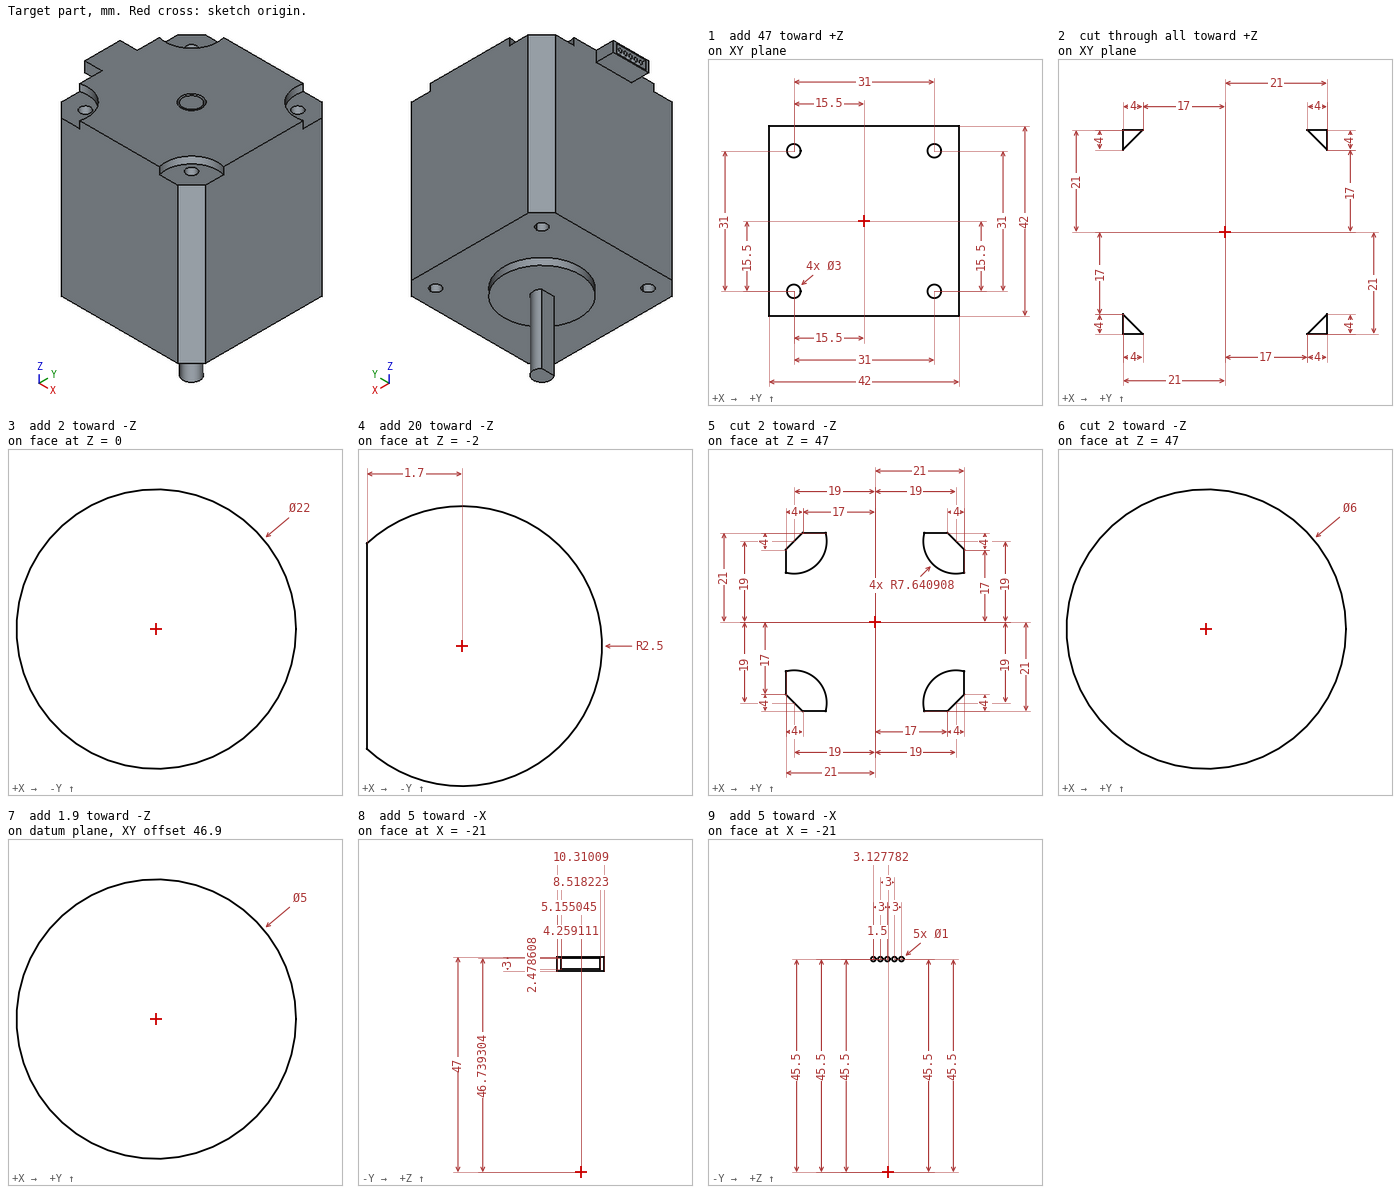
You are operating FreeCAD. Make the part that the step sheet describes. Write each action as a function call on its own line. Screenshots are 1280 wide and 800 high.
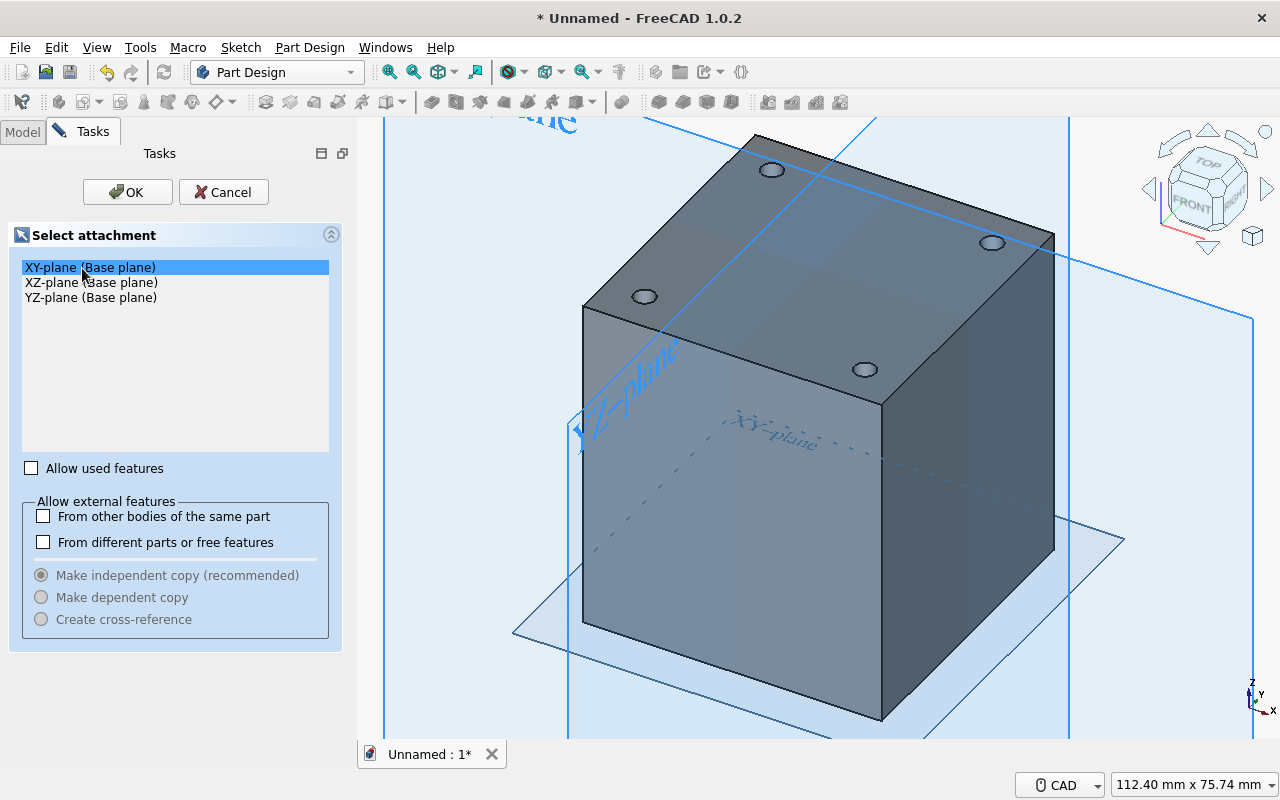
click(128, 192)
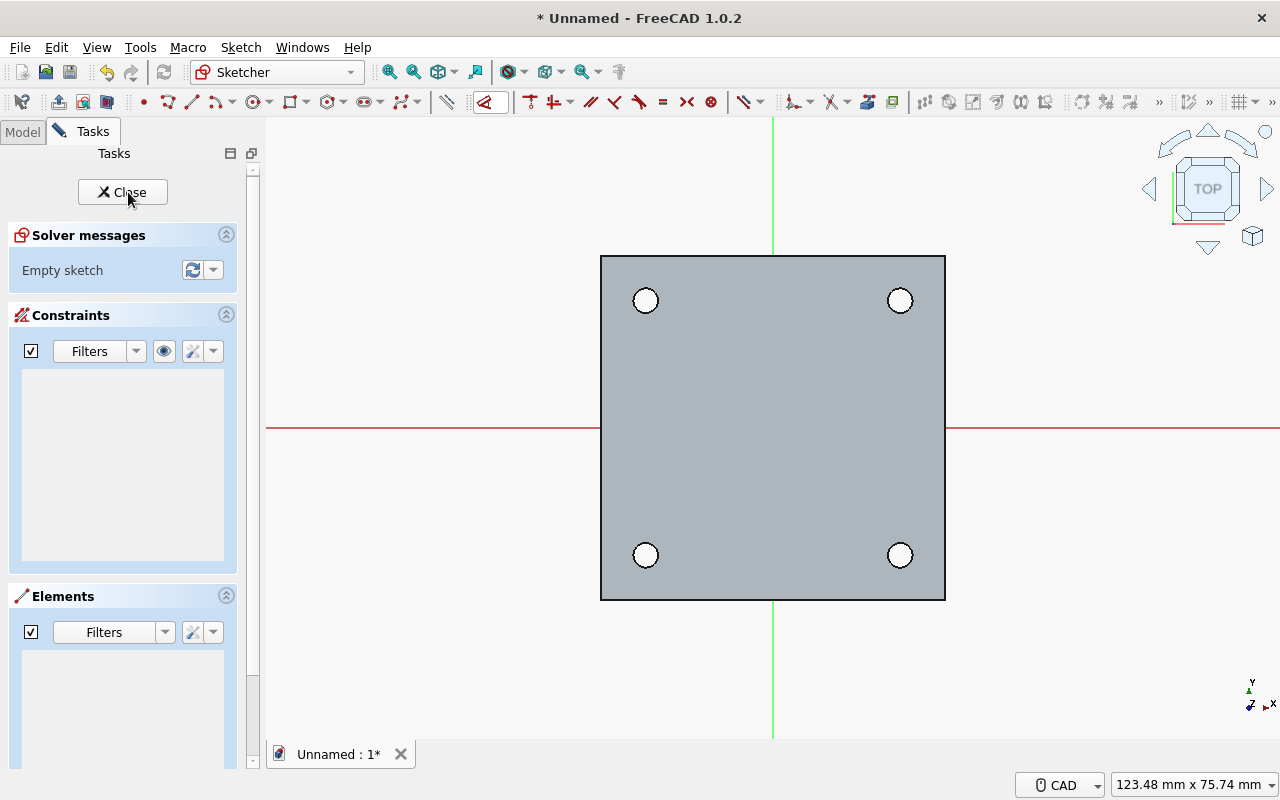
click(108, 102)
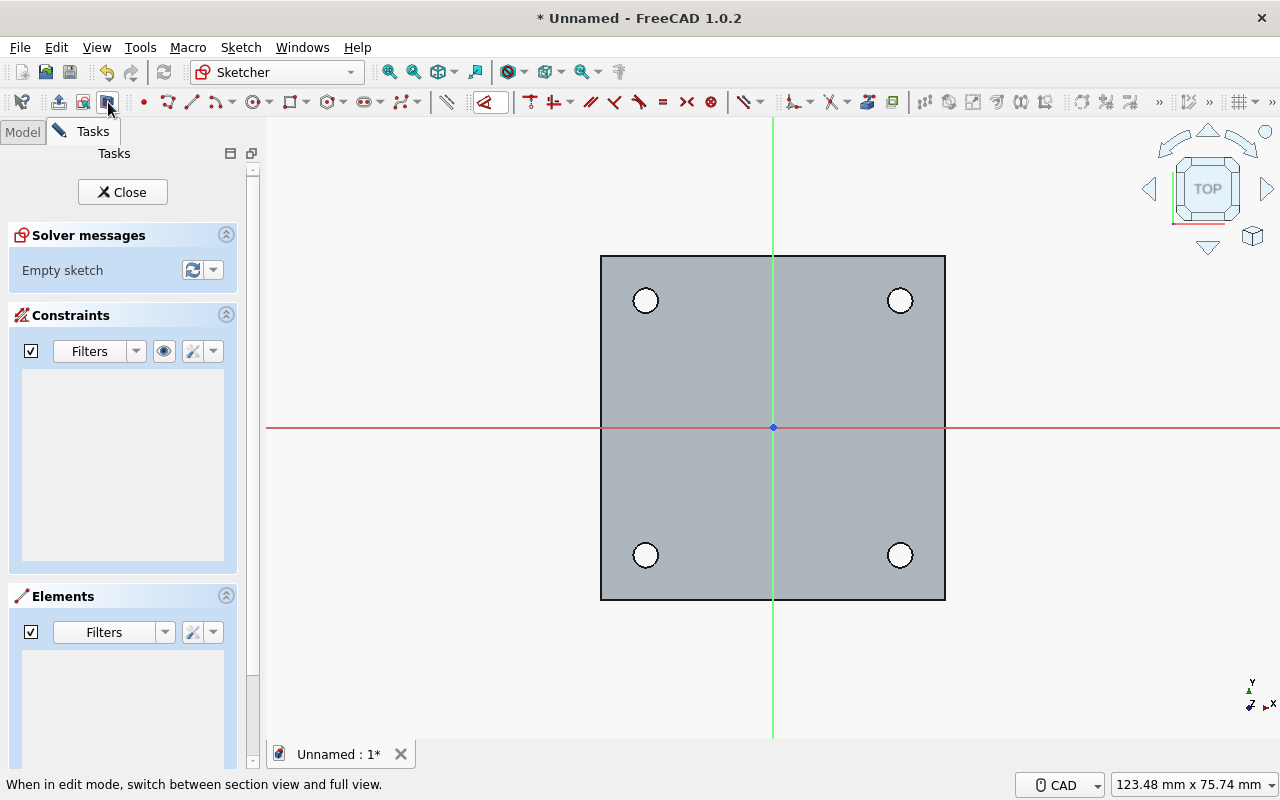
click(168, 102)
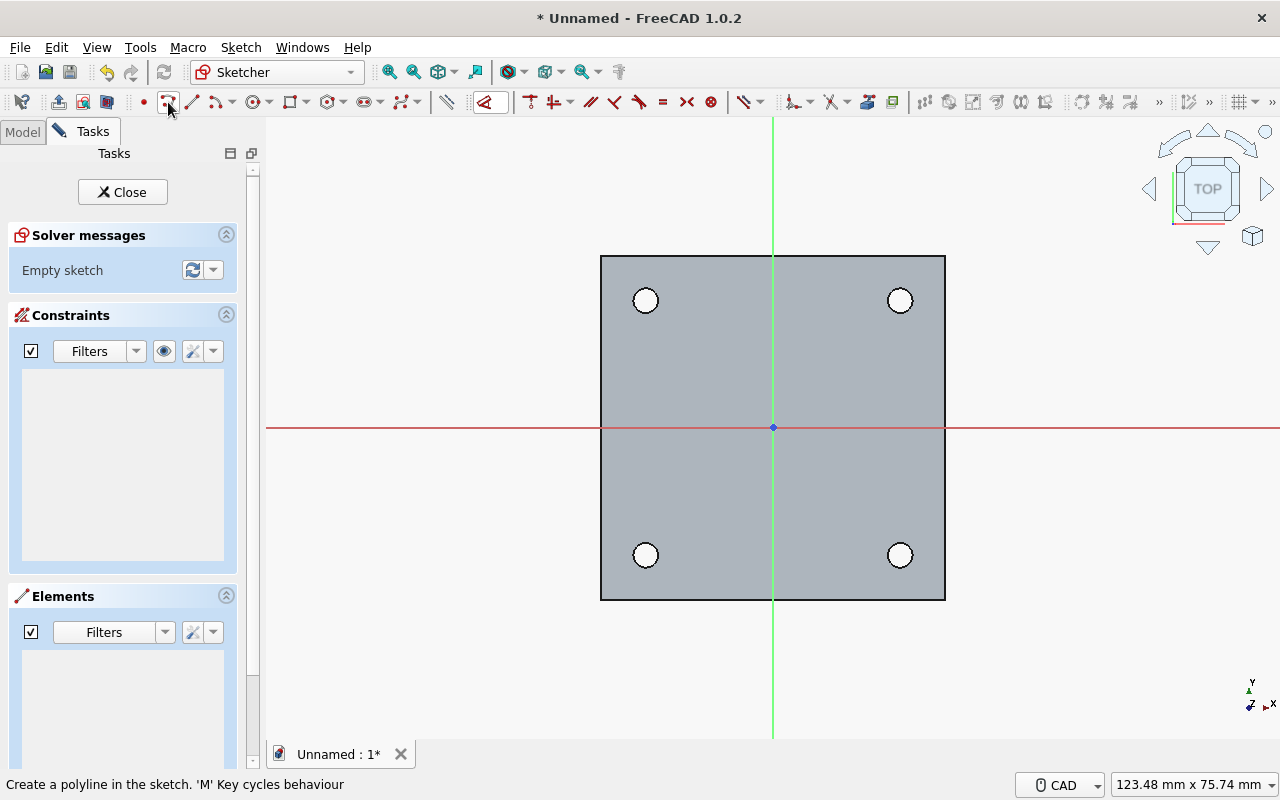
click(945, 288)
click(913, 256)
click(945, 256)
click(945, 289)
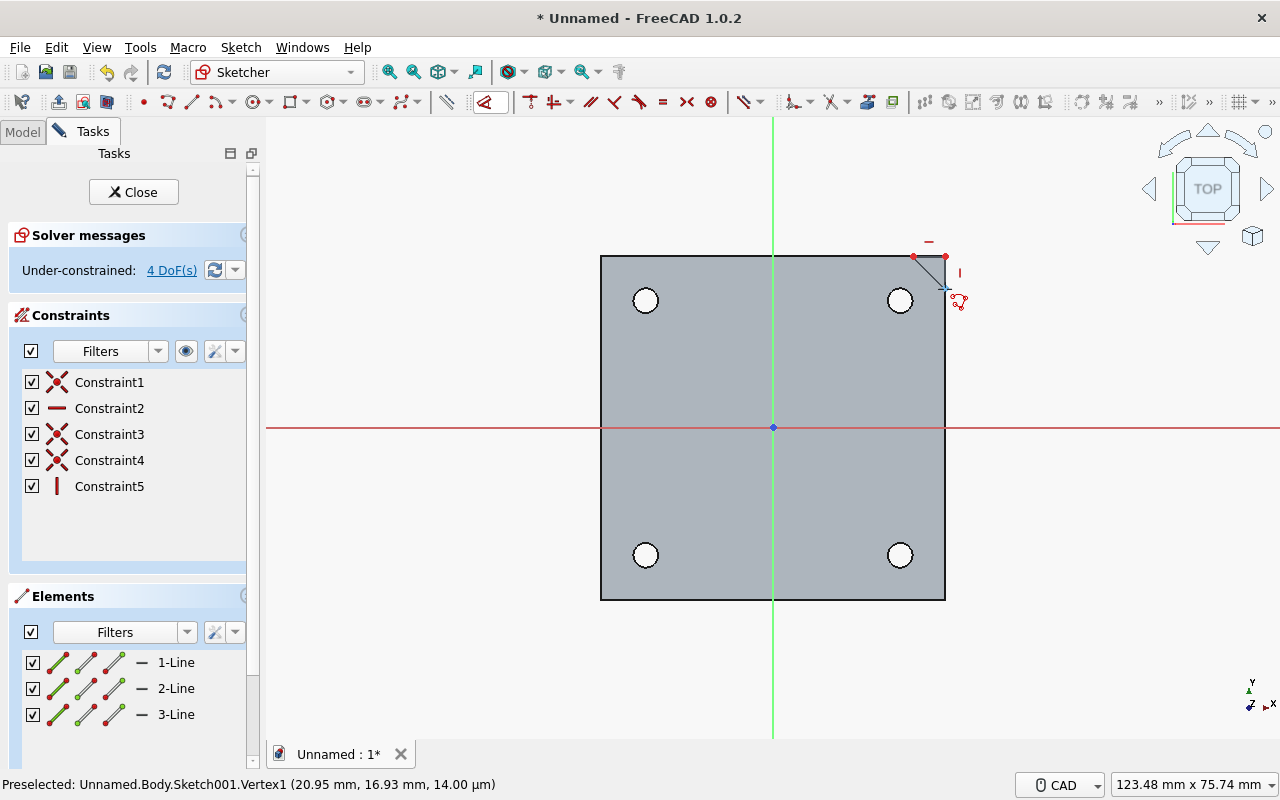
click(633, 256)
click(601, 288)
click(601, 256)
click(633, 257)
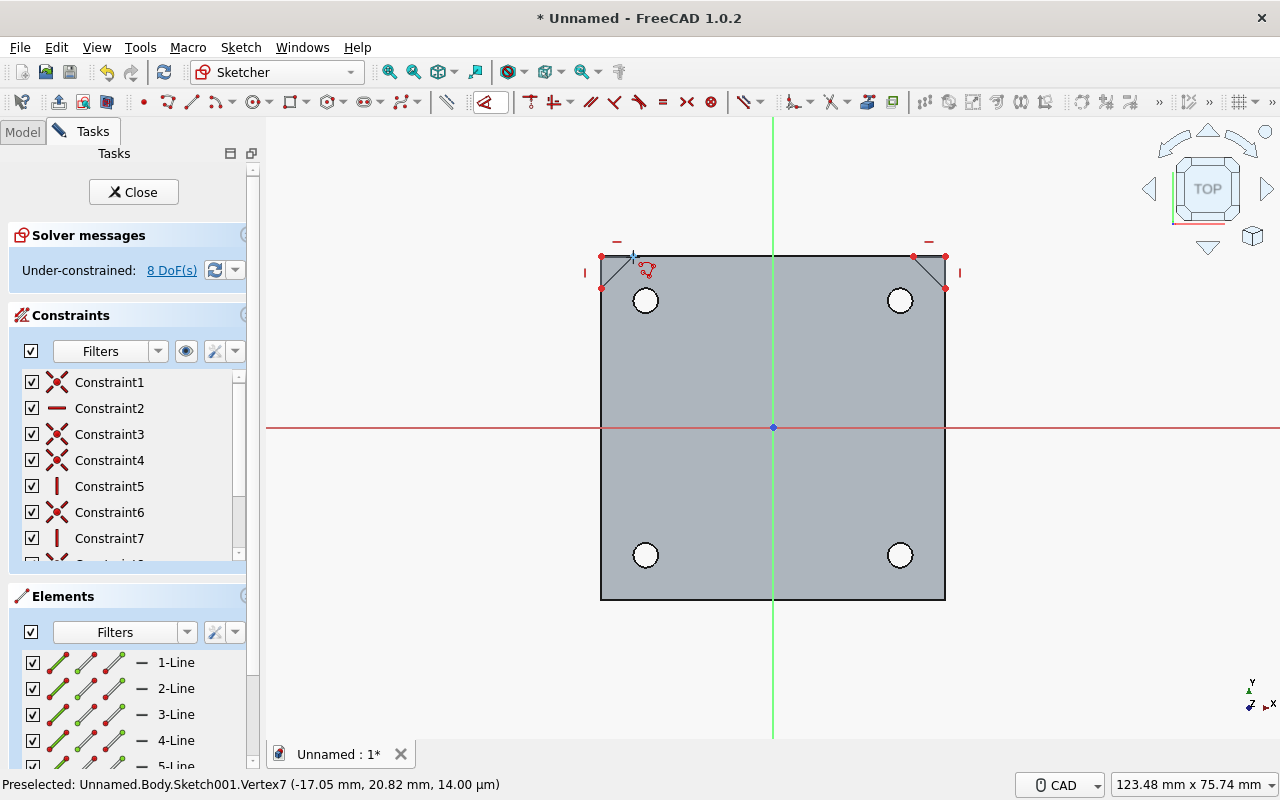
click(601, 568)
click(633, 600)
click(601, 600)
click(601, 569)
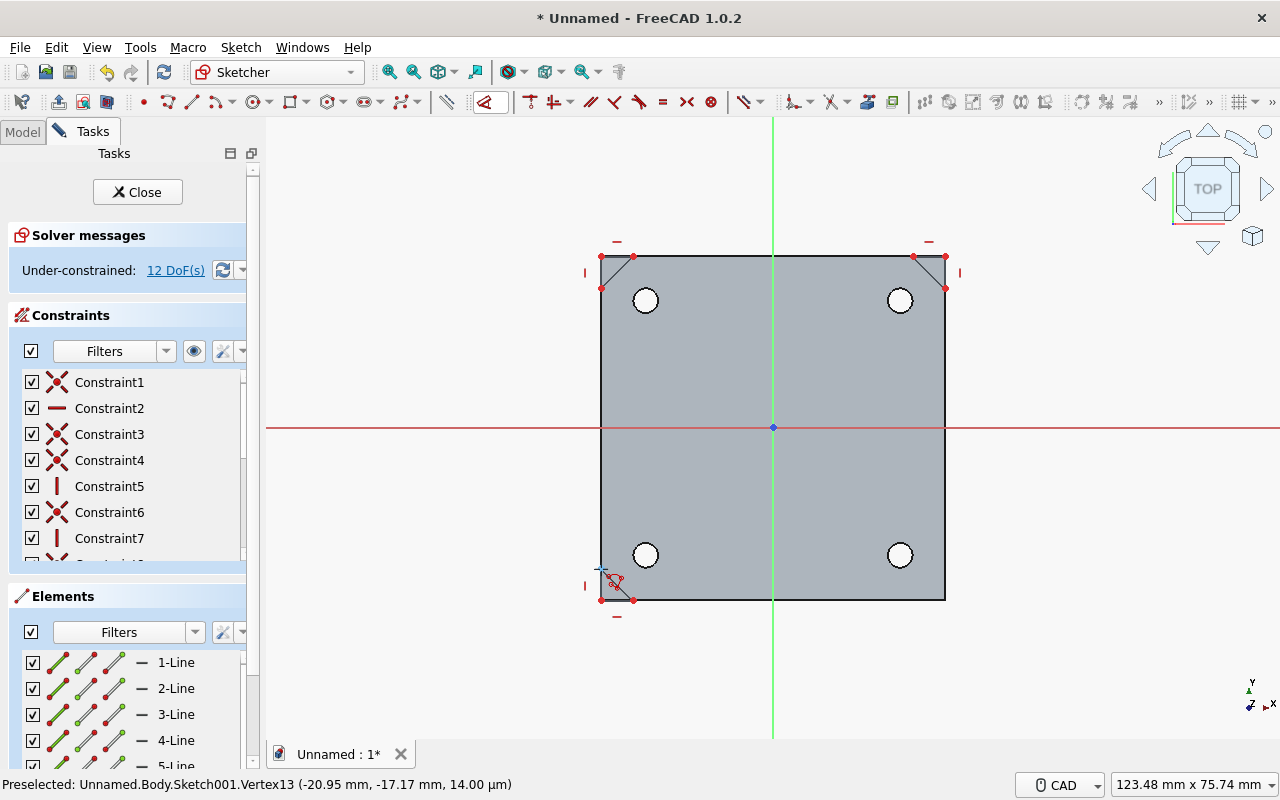
click(913, 600)
click(945, 568)
click(945, 600)
click(913, 601)
key(Escape)
key(Escape)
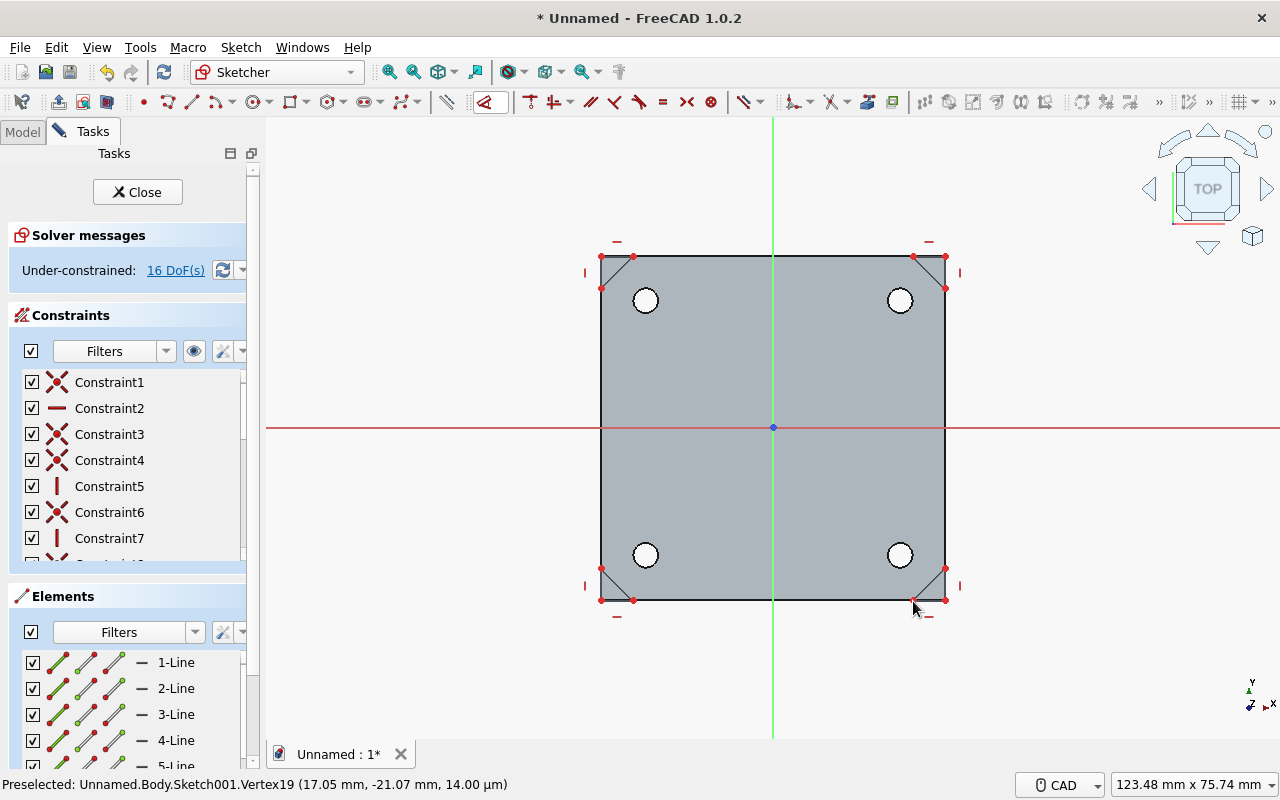
scroll(935, 257, up, 2)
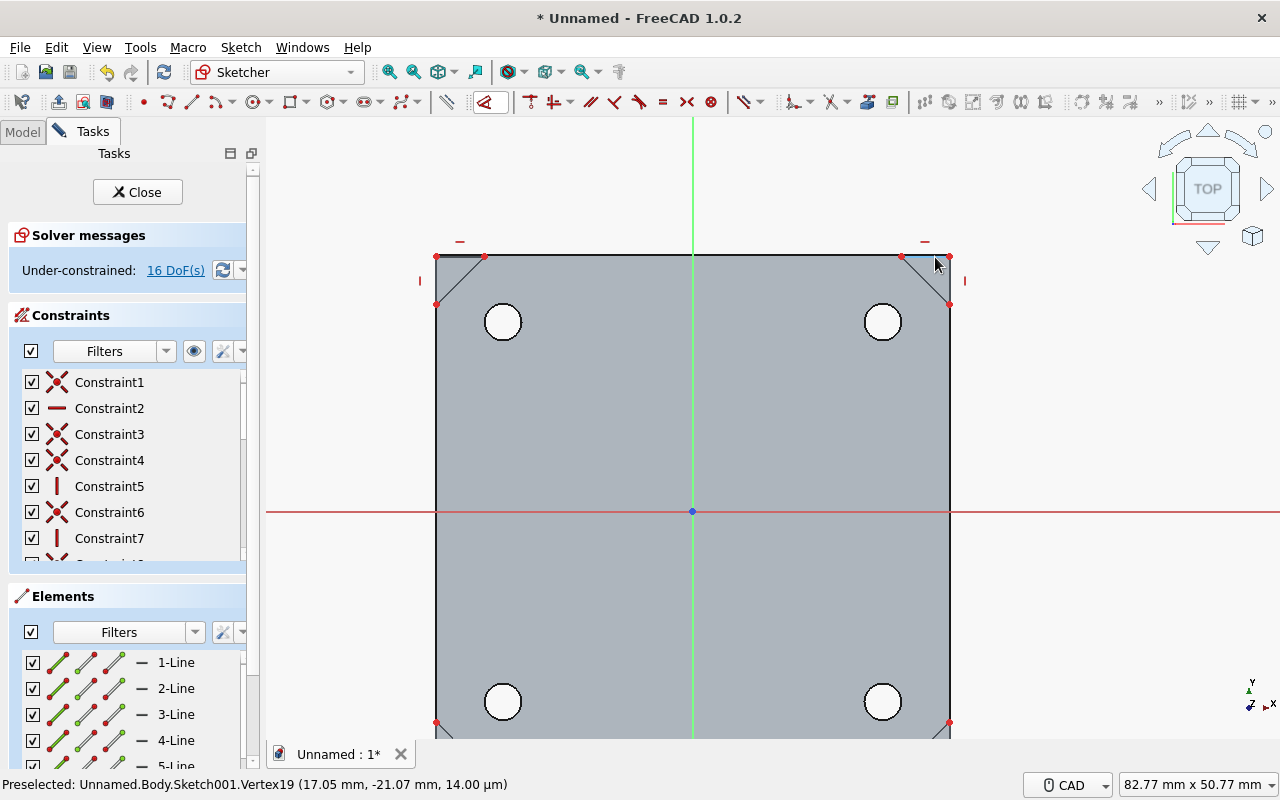
click(935, 257)